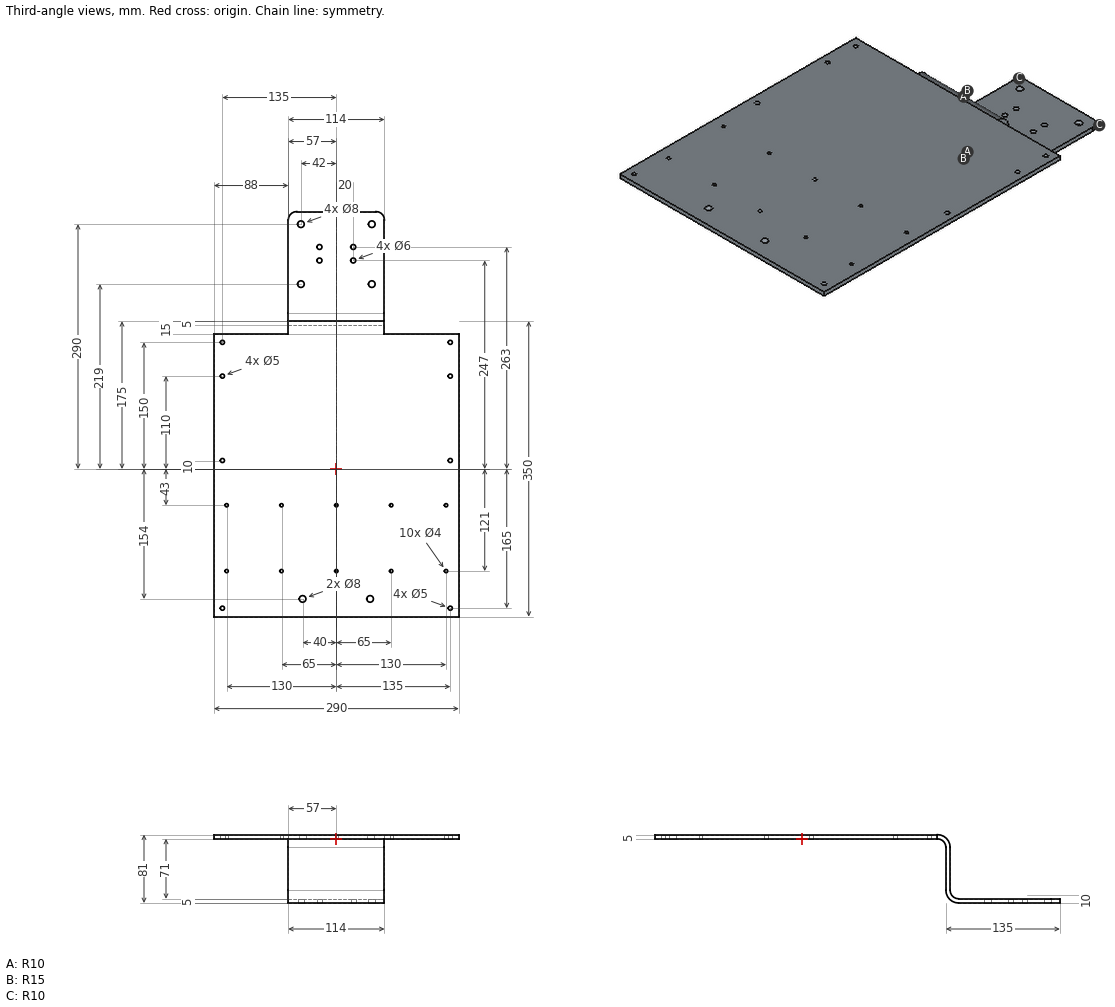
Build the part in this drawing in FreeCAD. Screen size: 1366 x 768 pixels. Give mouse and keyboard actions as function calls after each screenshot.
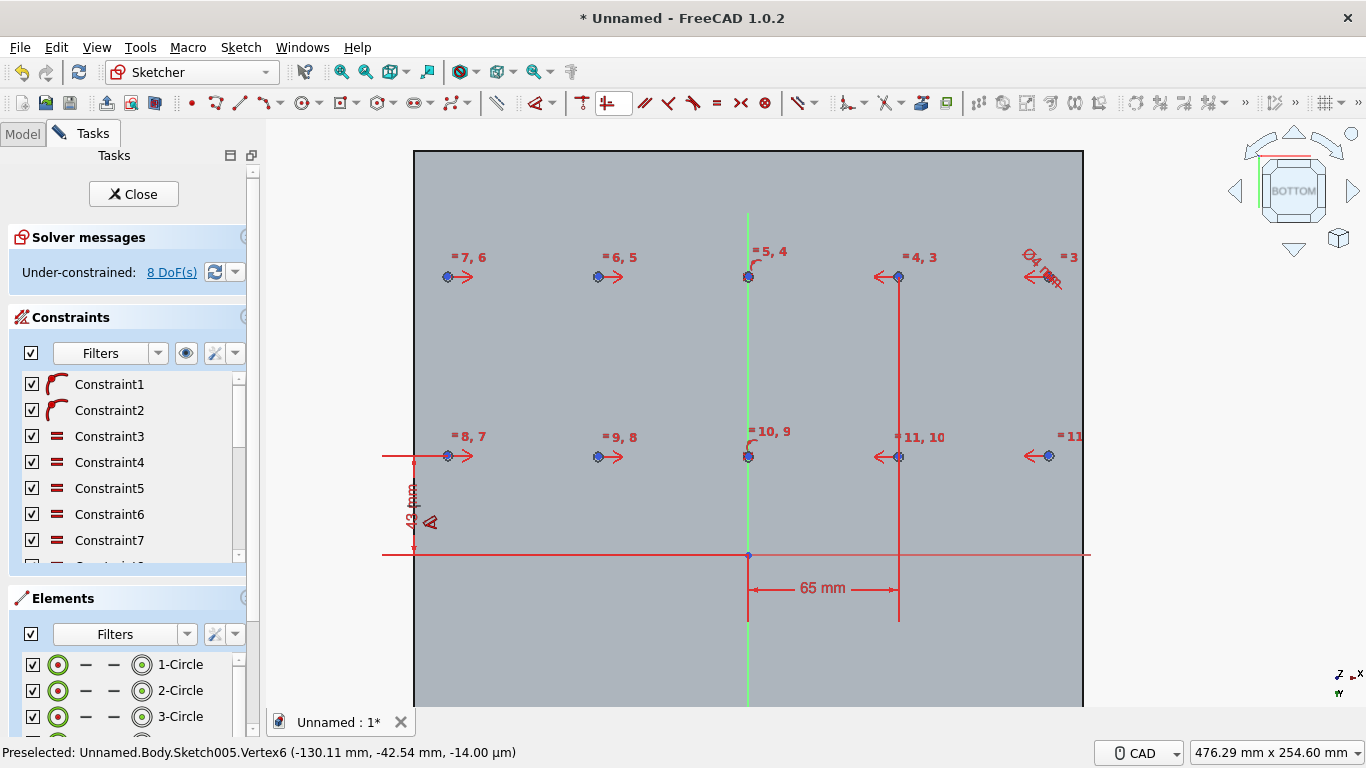
click(598, 457)
click(673, 589)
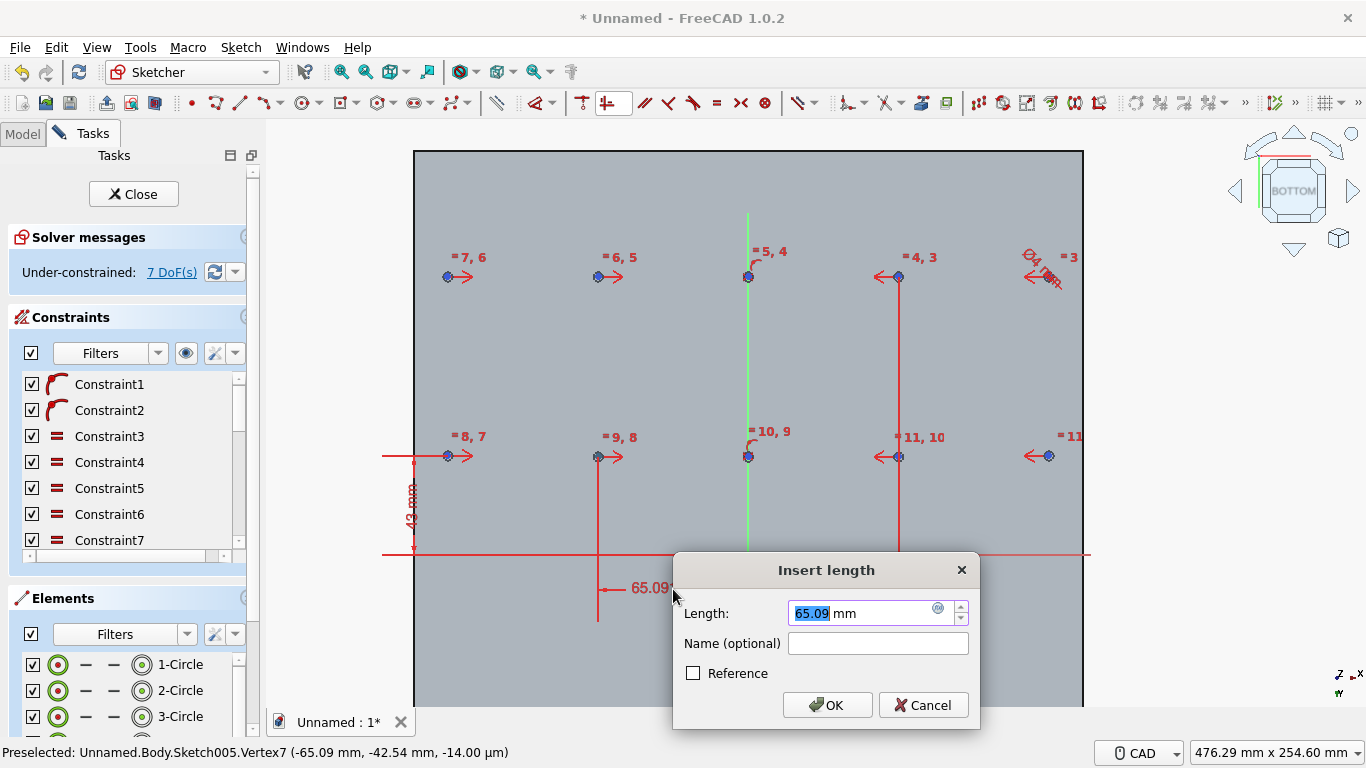
text(65)
key(Return)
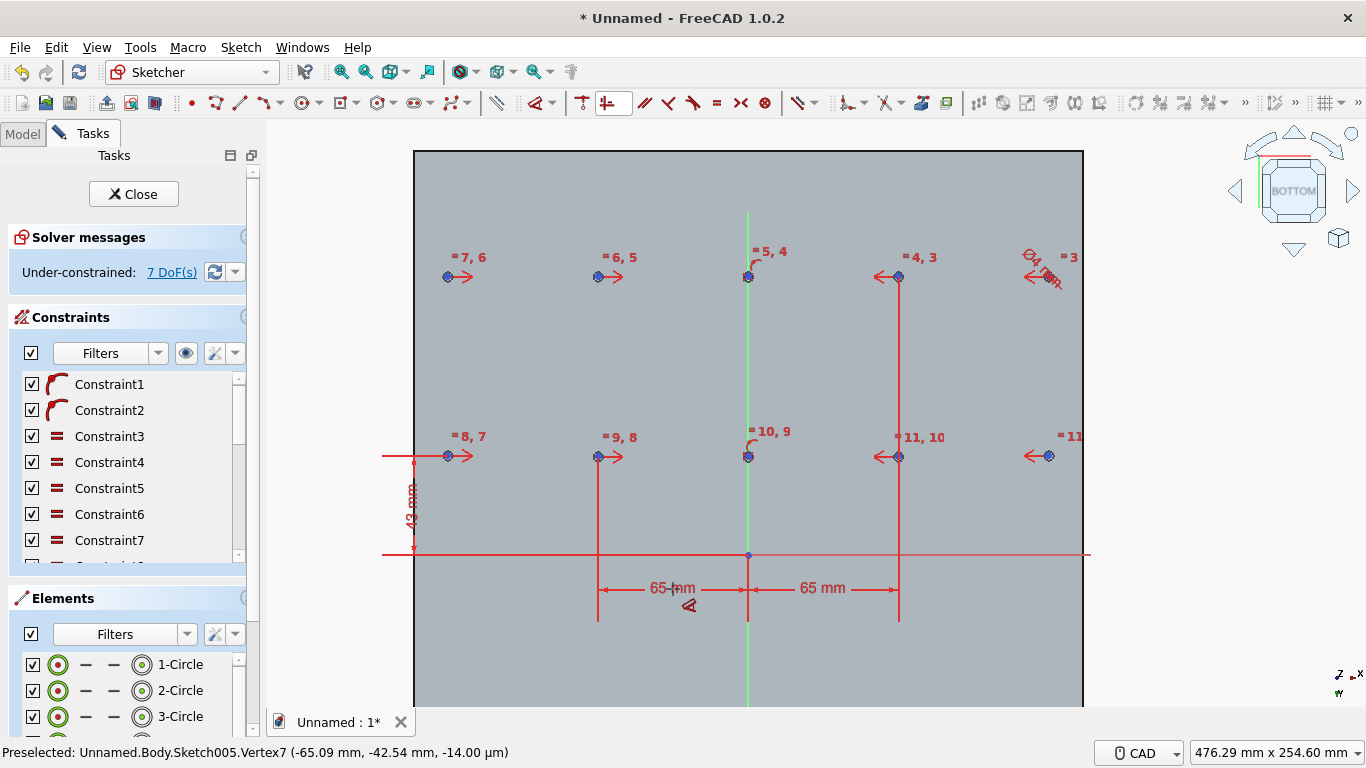
click(598, 457)
click(564, 506)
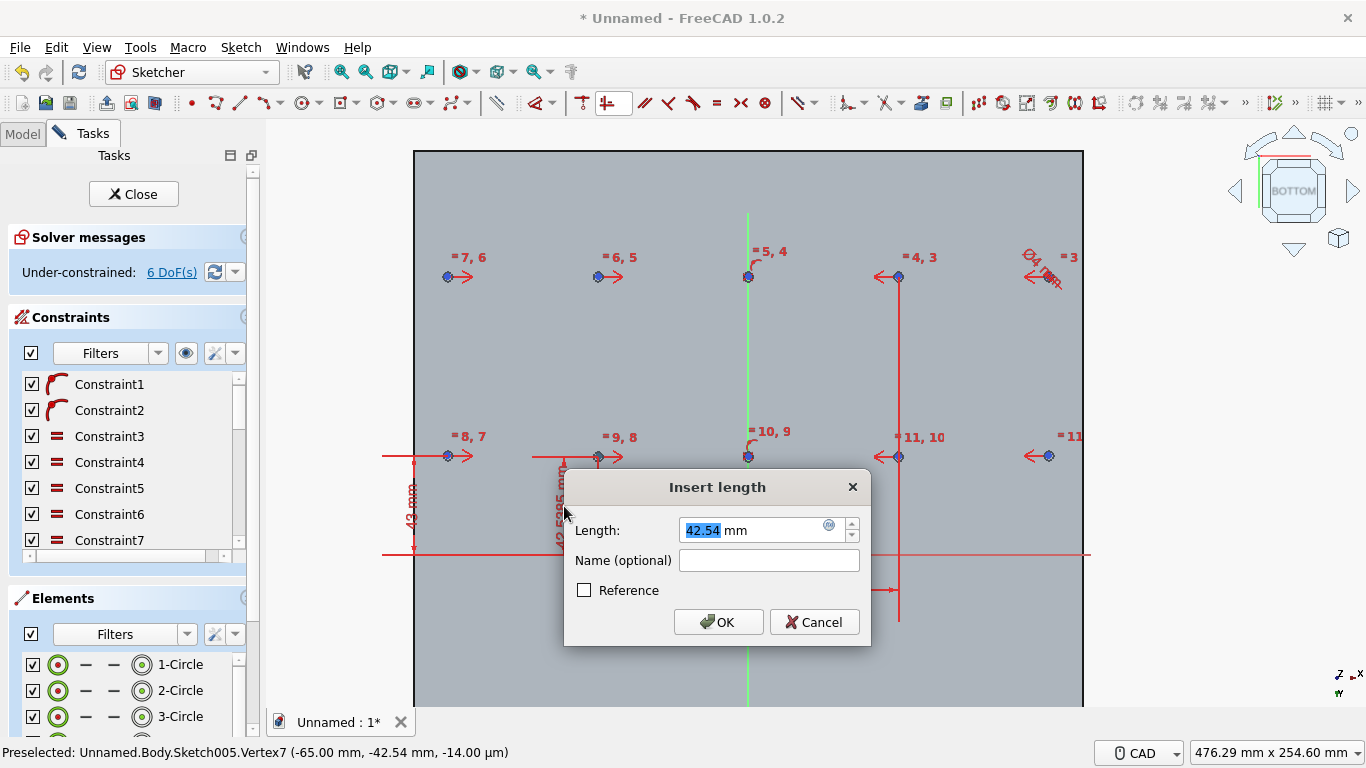
text(43)
key(Return)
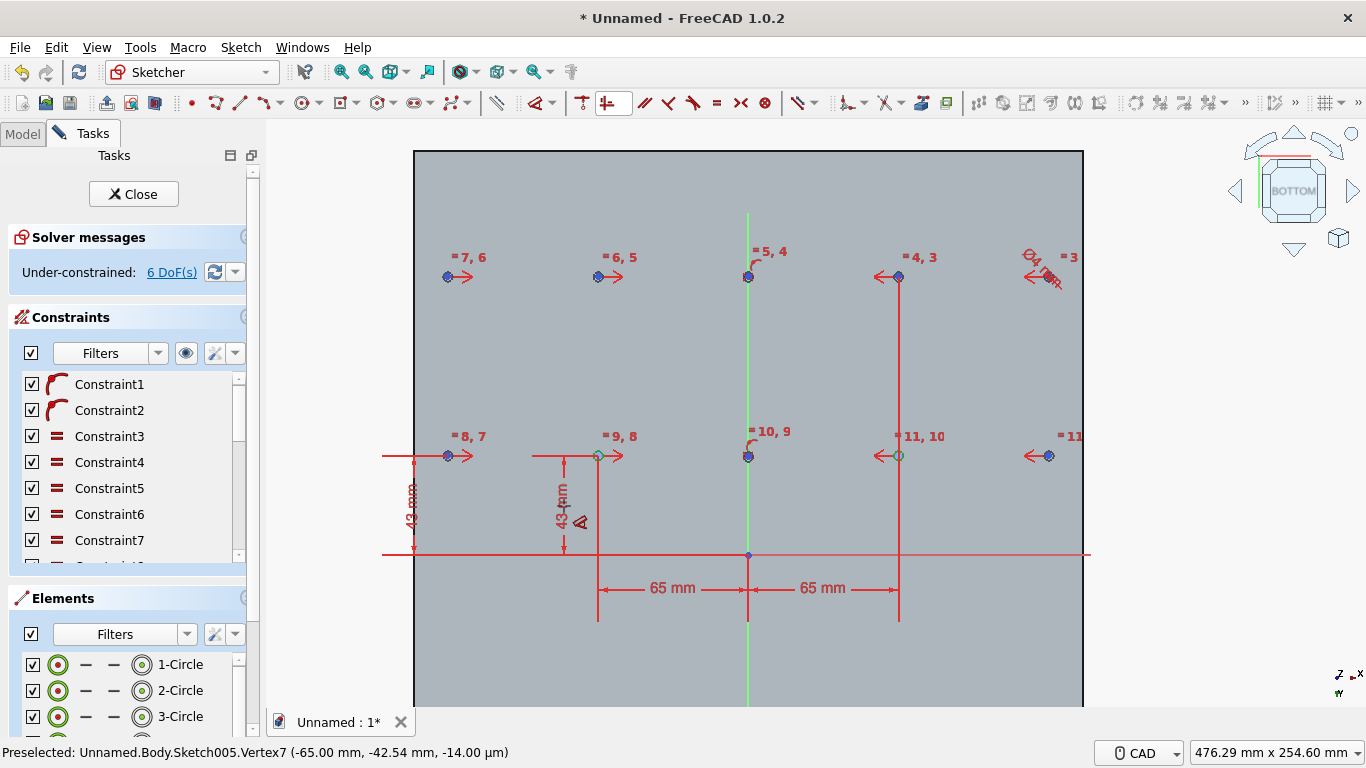
click(748, 457)
click(782, 506)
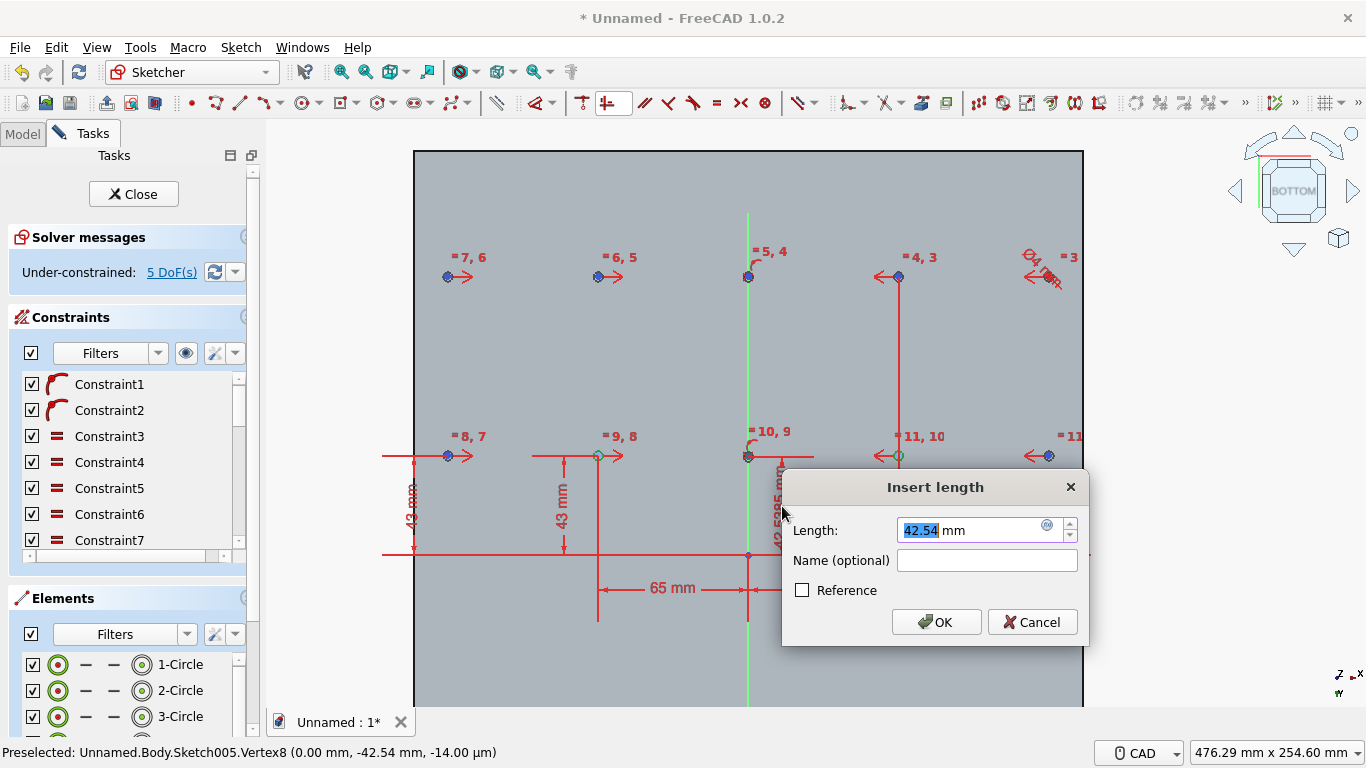
text(43)
key(Return)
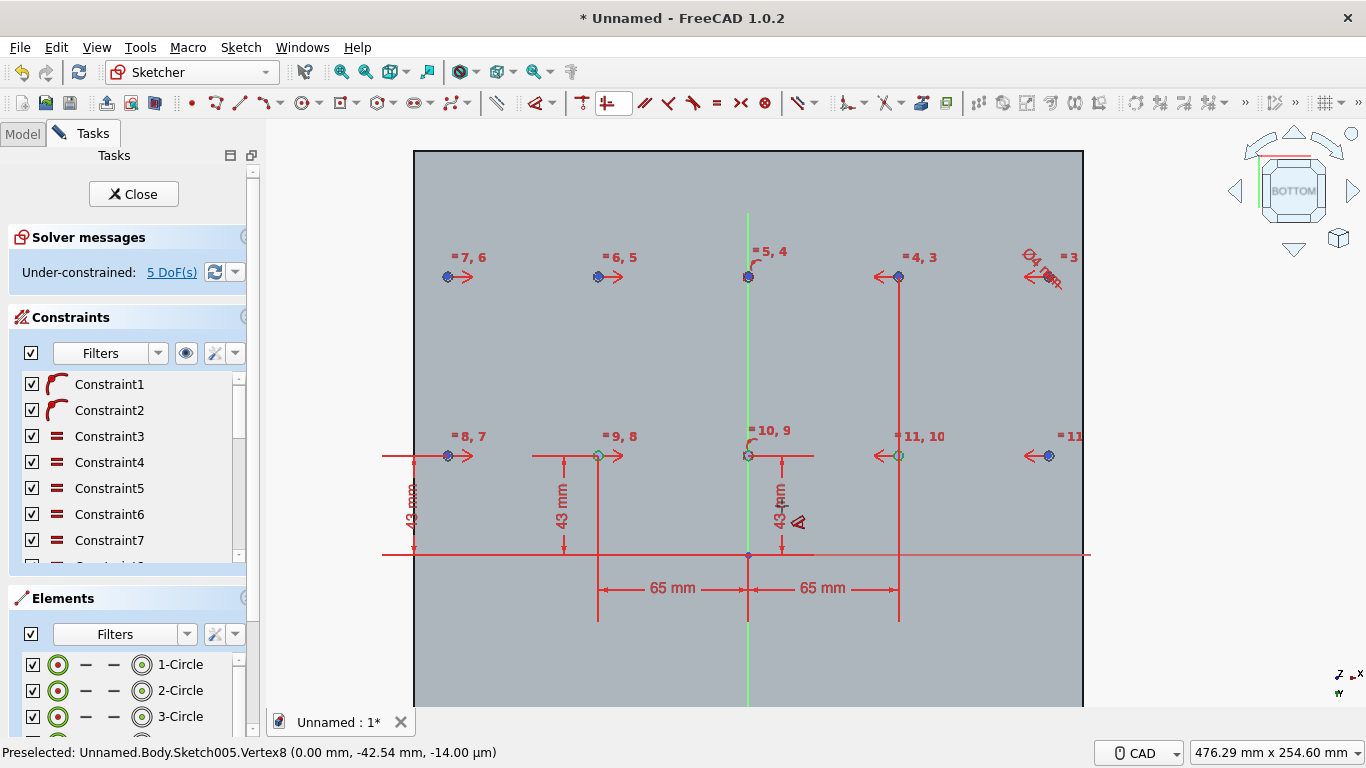
click(1049, 277)
click(899, 589)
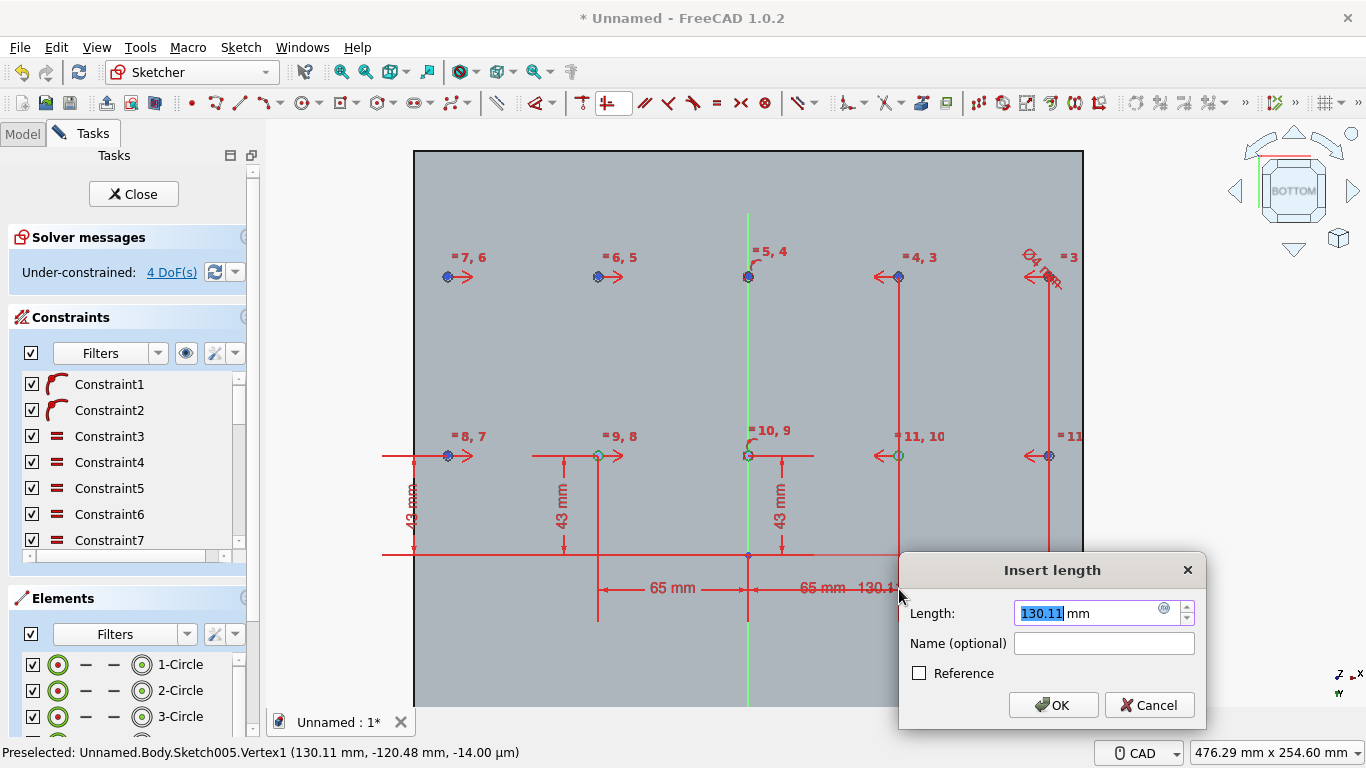
text(130)
key(Return)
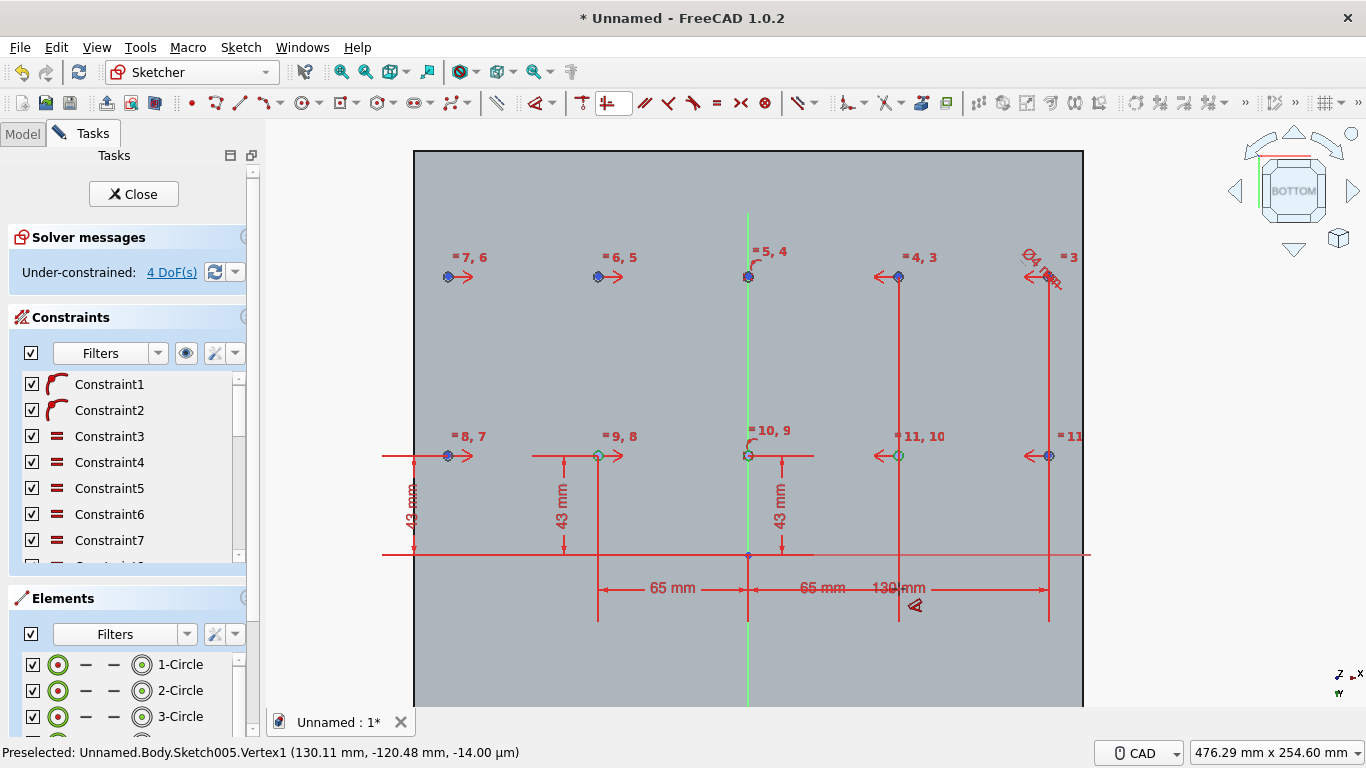
click(1049, 277)
click(1083, 416)